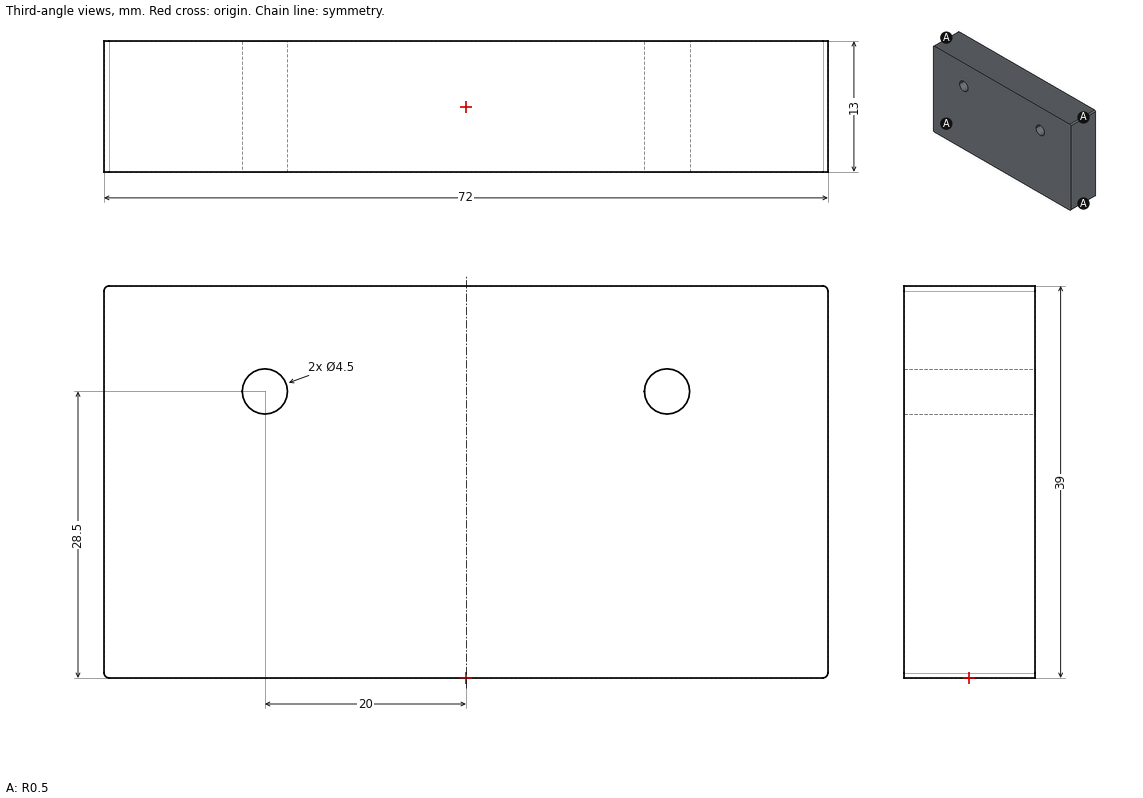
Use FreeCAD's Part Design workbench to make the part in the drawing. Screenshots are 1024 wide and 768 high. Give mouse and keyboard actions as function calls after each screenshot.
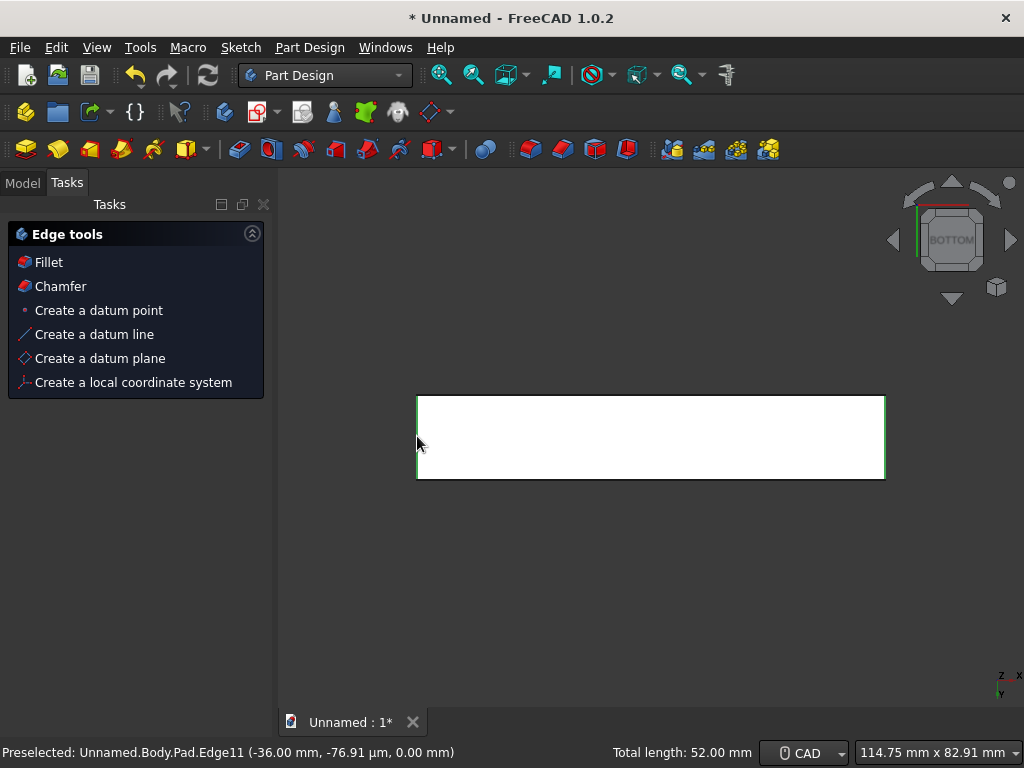
click(532, 150)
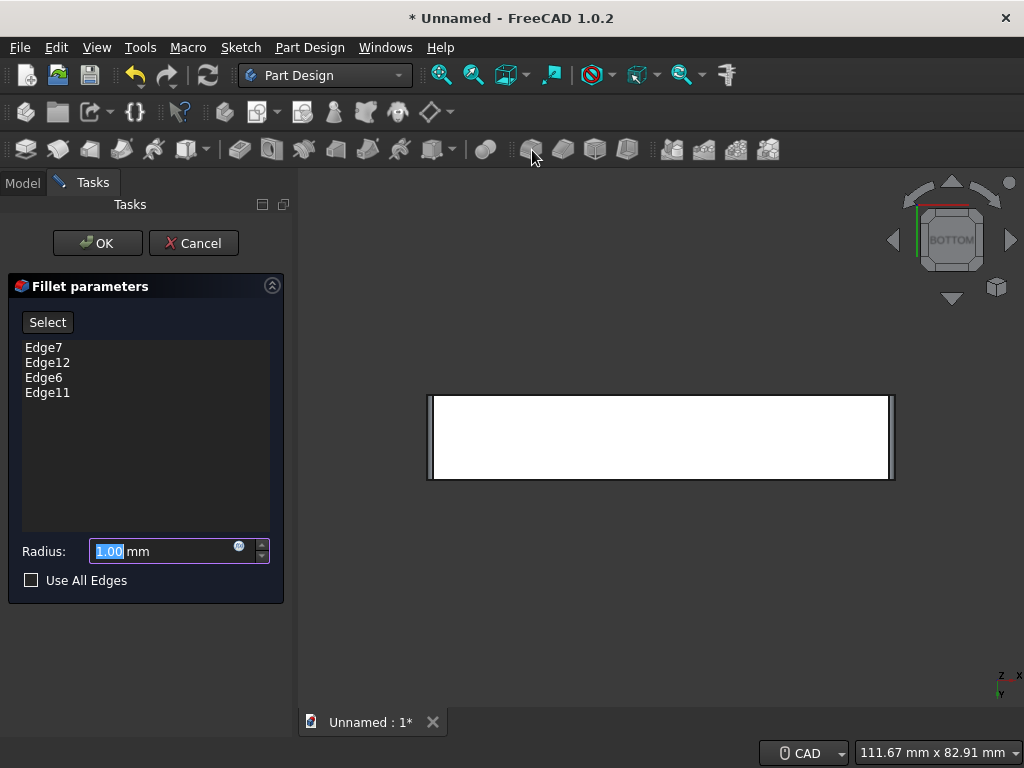
text(0.5)
key(Tab)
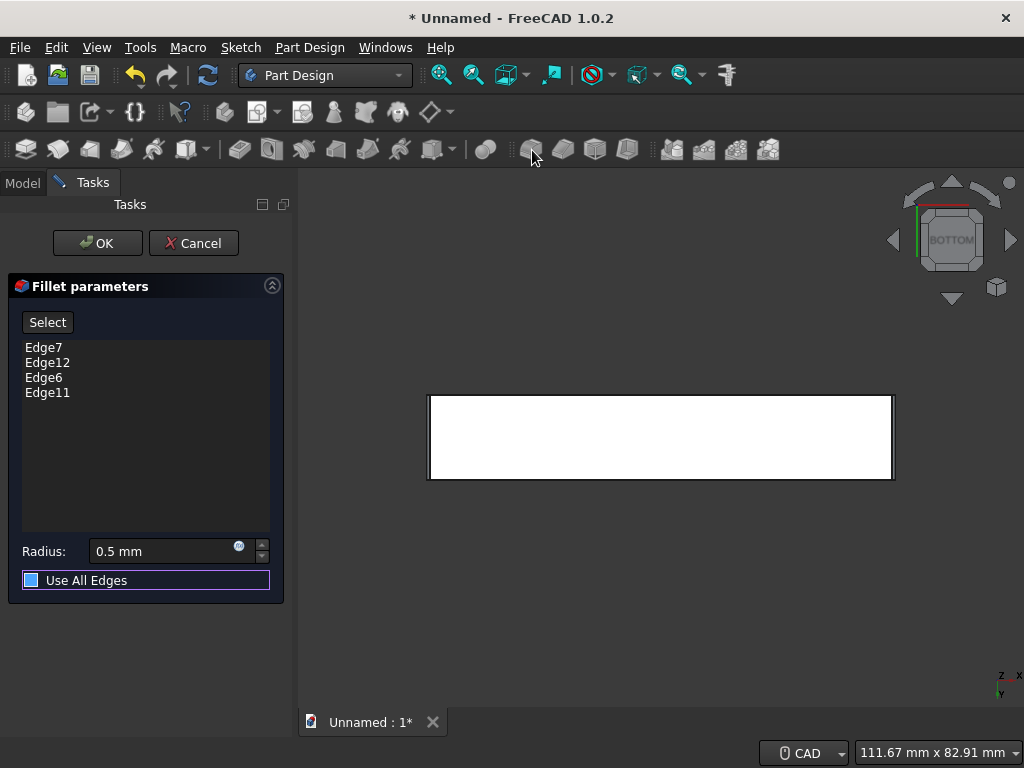
click(98, 243)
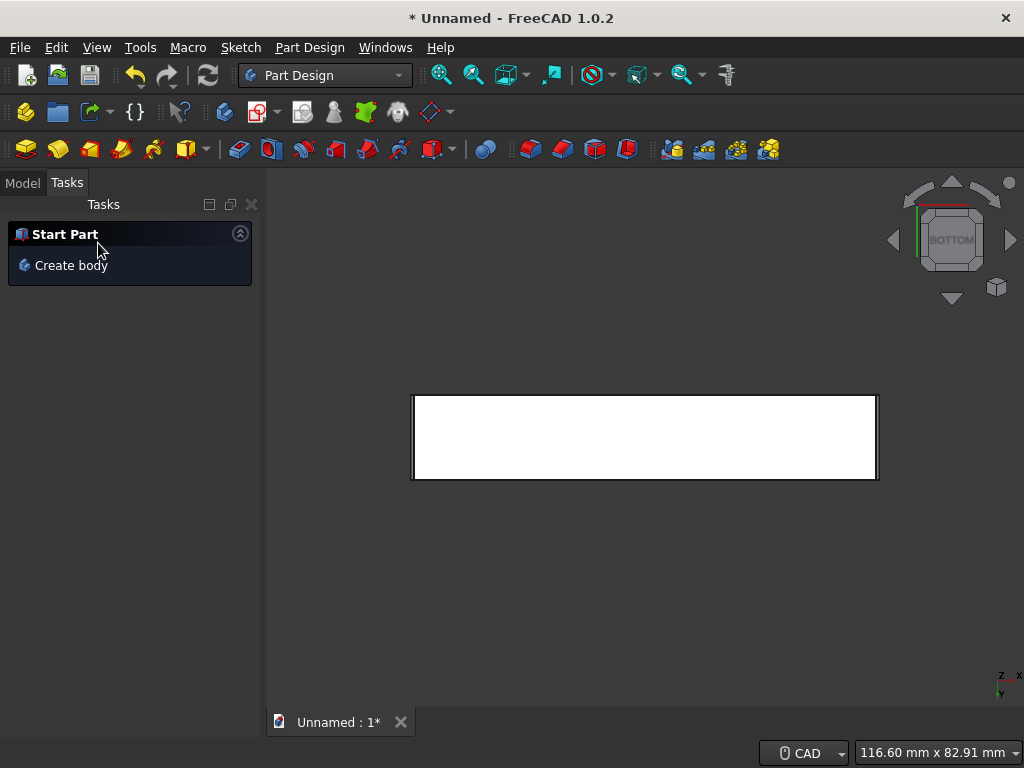
key(4)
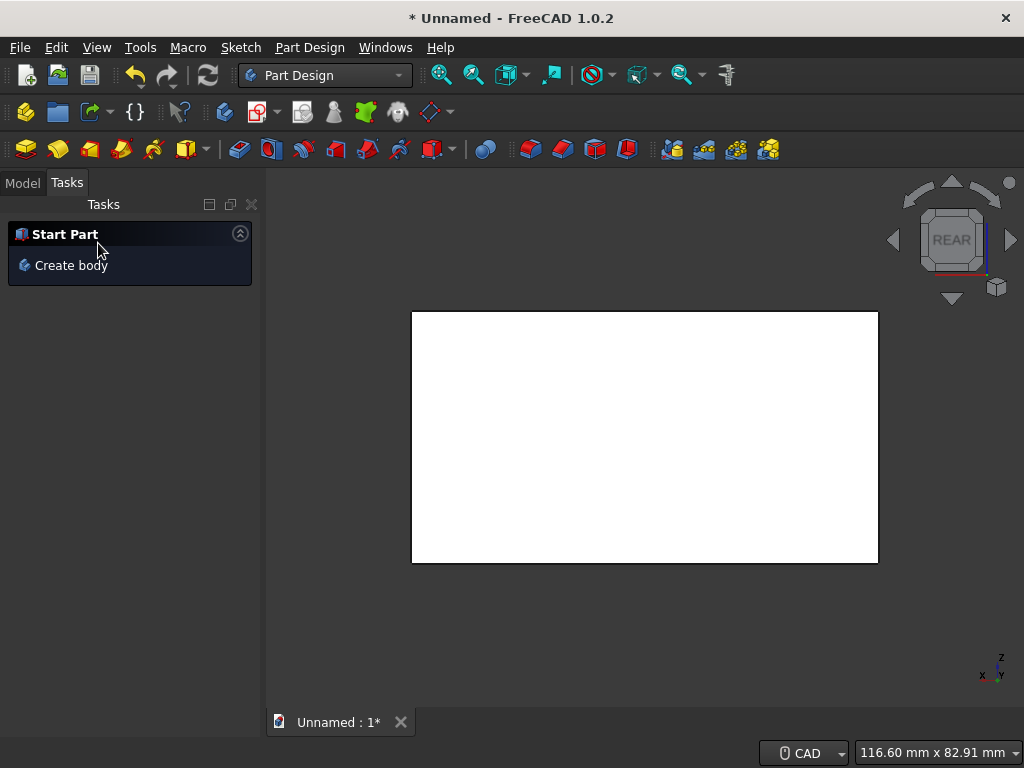
click(578, 436)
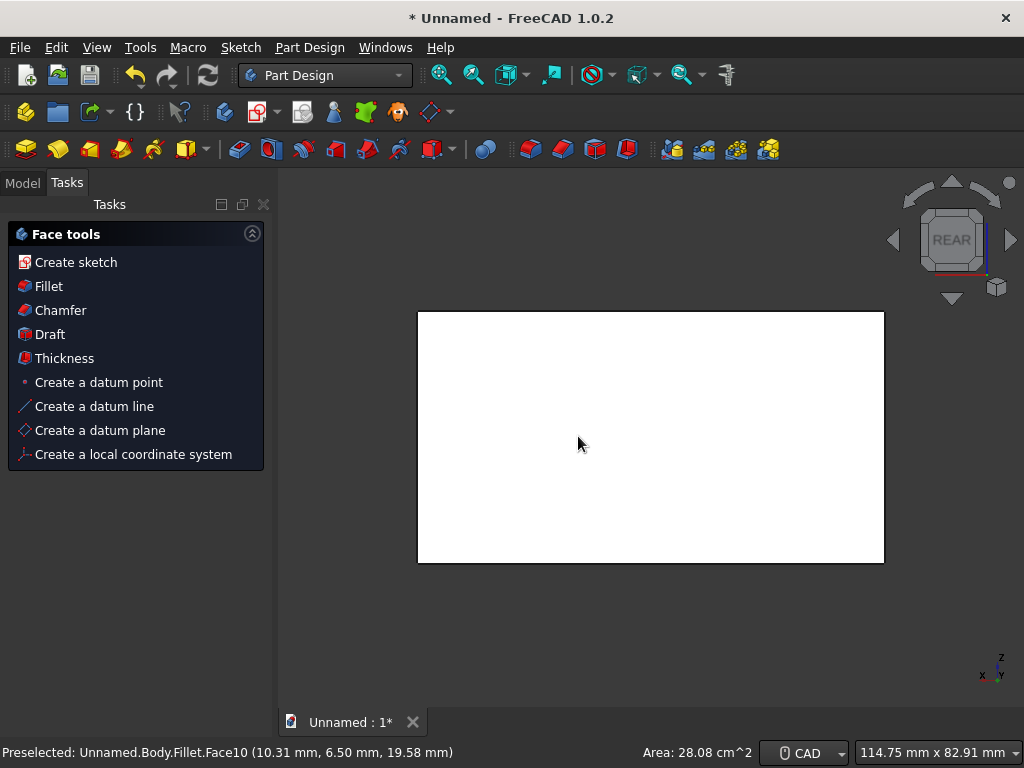
click(258, 112)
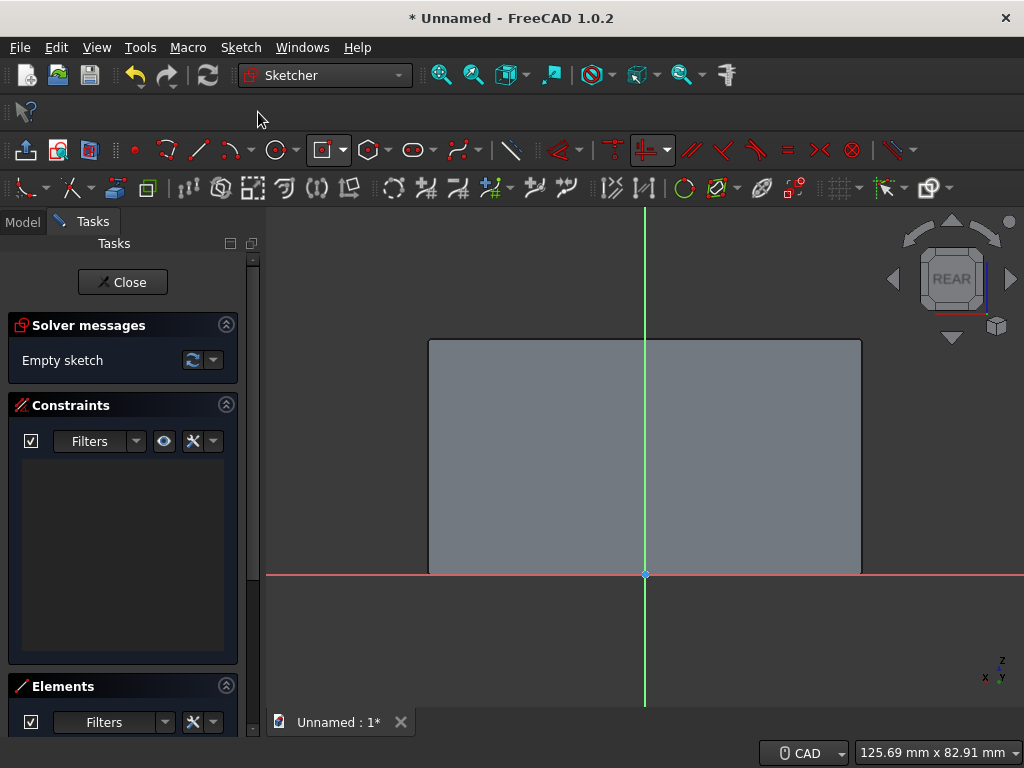
scroll(784, 532, up, 2)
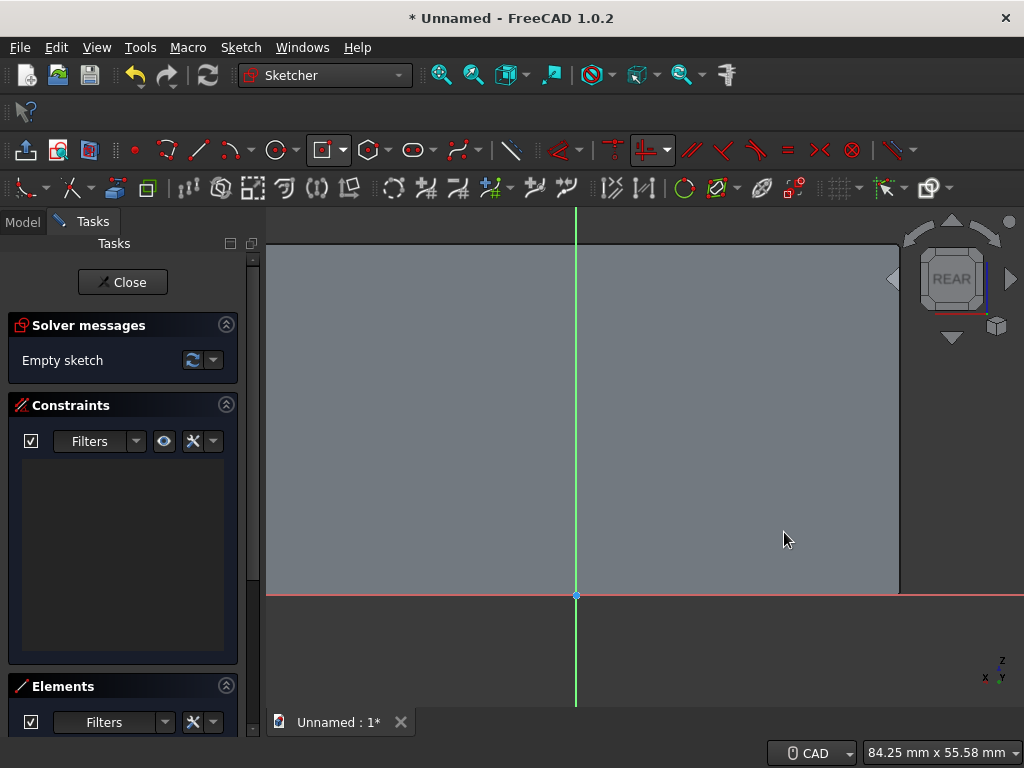
click(276, 150)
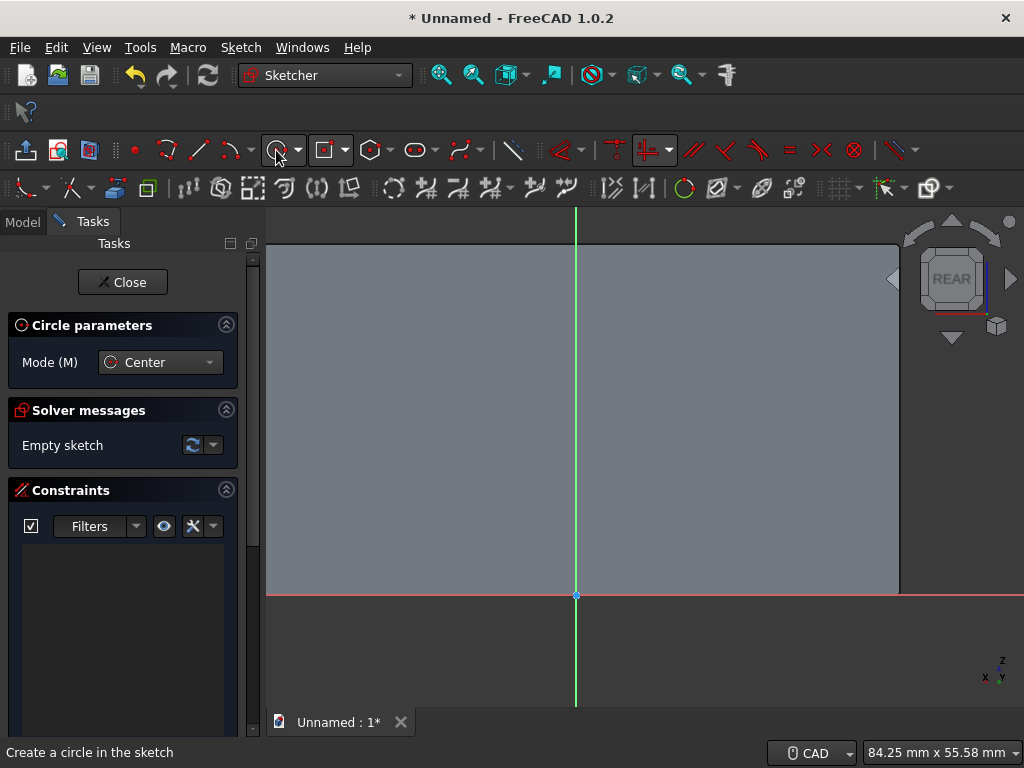
click(756, 339)
click(771, 325)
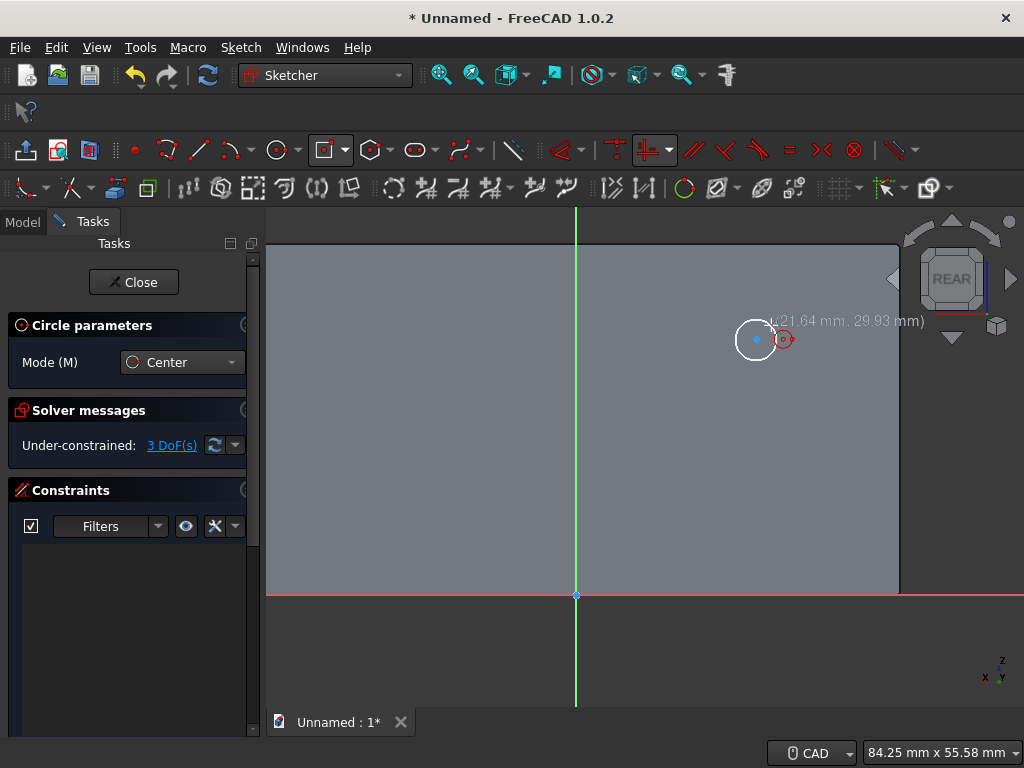
click(396, 339)
click(411, 325)
key(Escape)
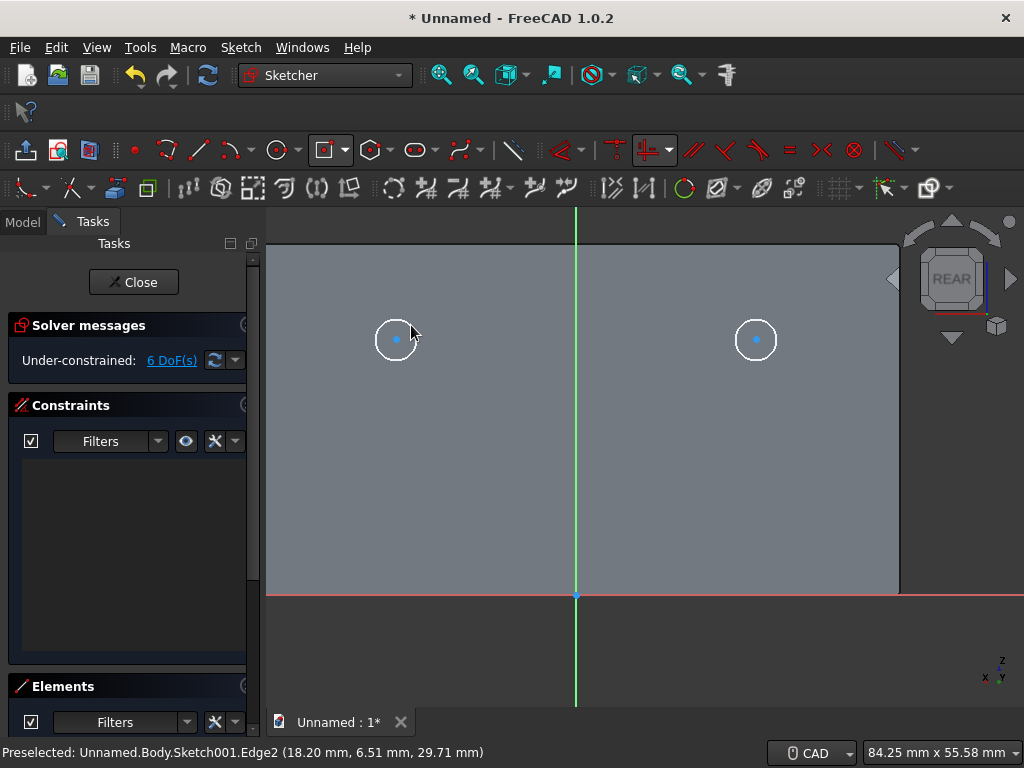
click(770, 325)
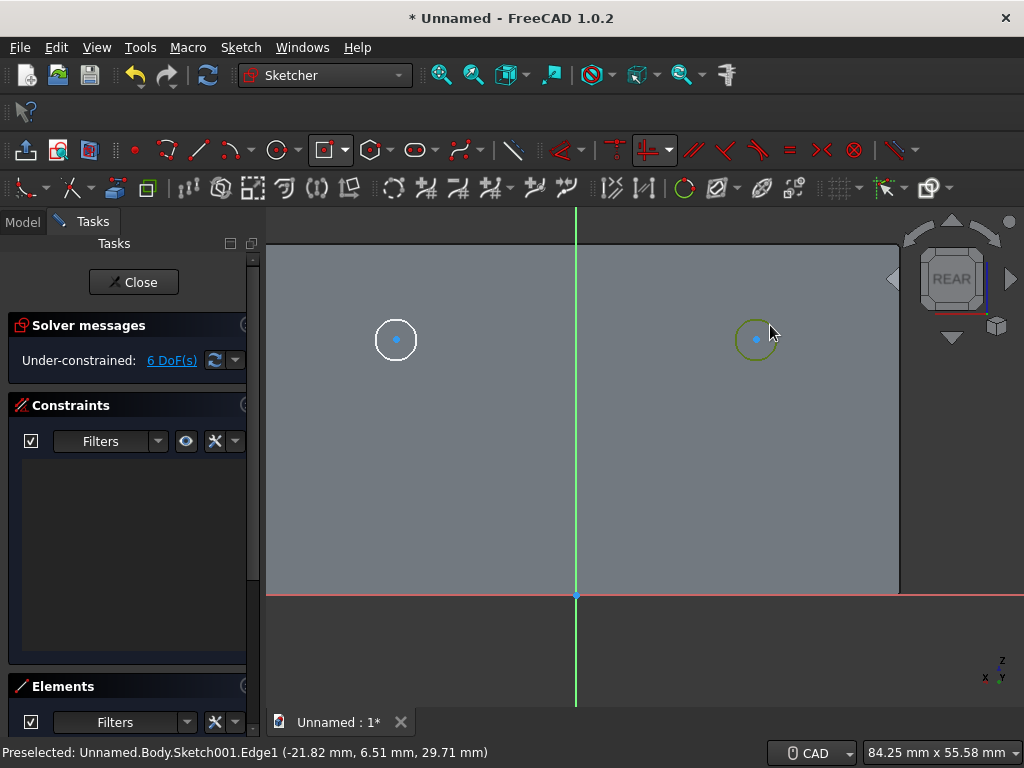
click(410, 325)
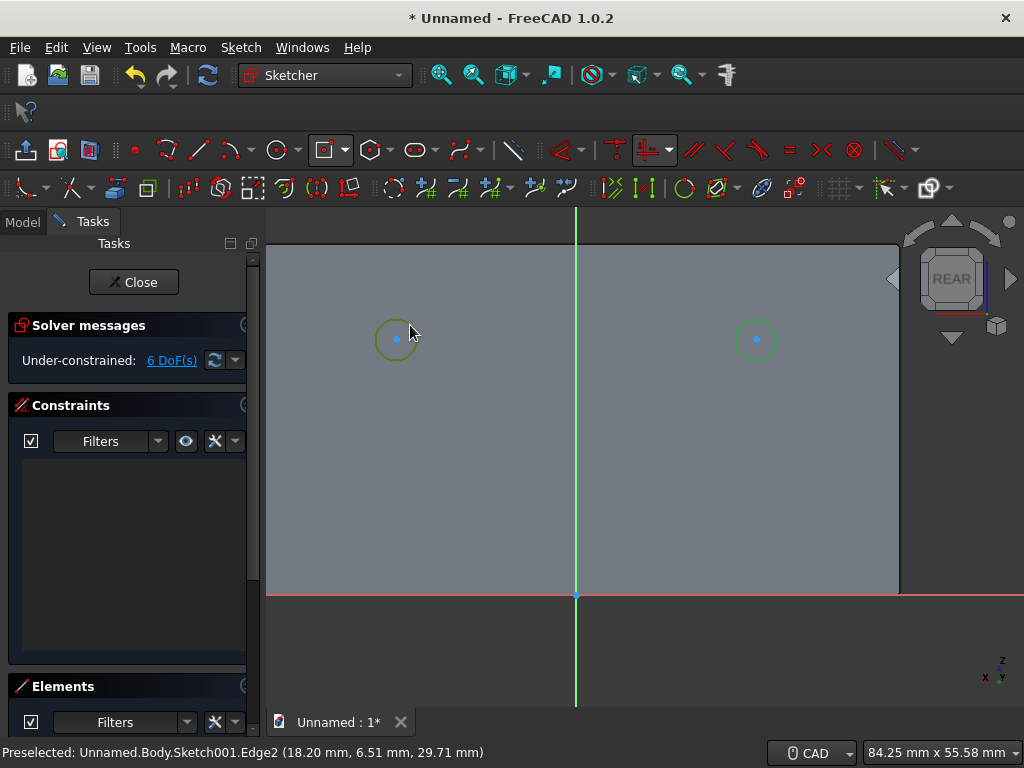
click(790, 150)